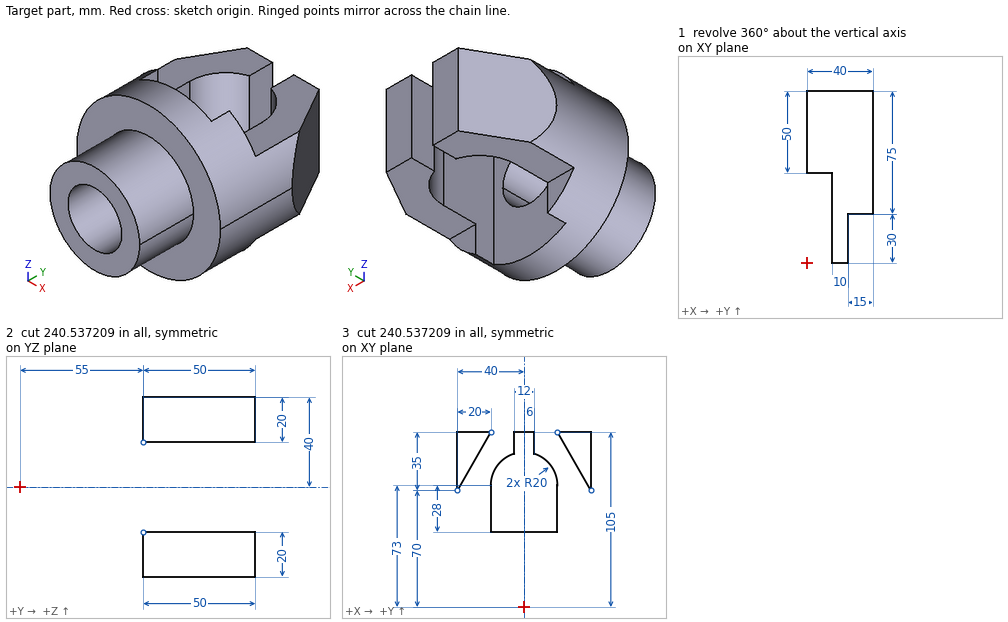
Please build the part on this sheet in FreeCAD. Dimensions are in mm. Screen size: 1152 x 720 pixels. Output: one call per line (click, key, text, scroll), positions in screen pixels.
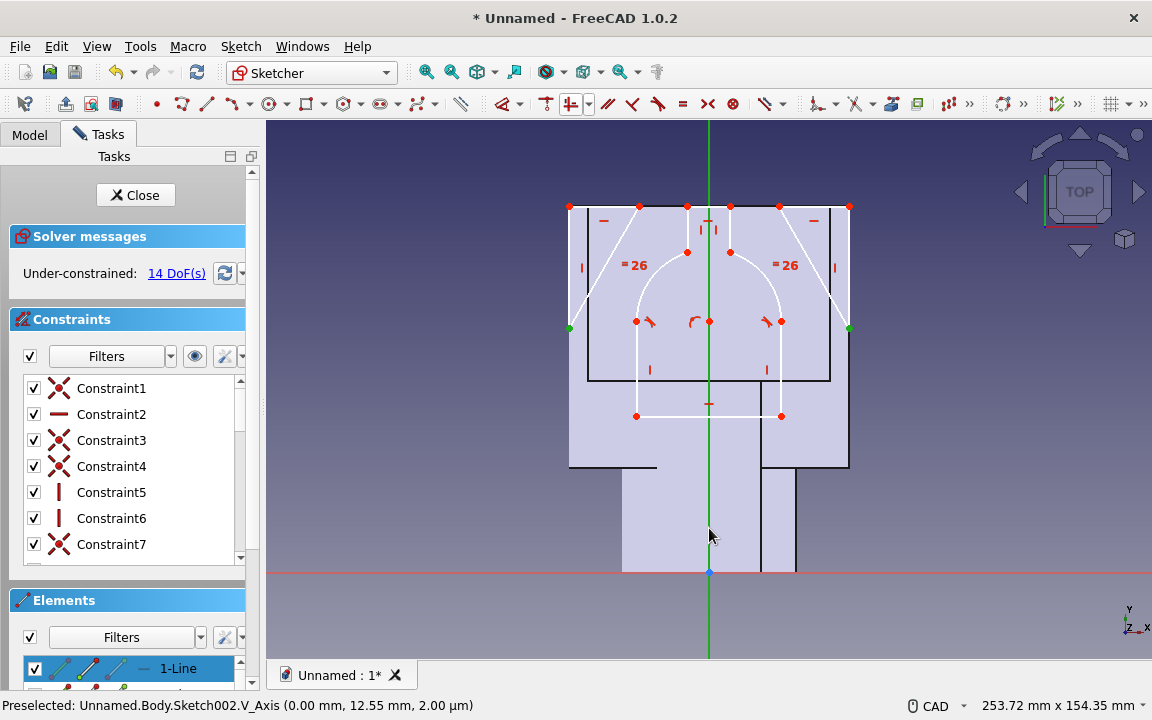
click(708, 104)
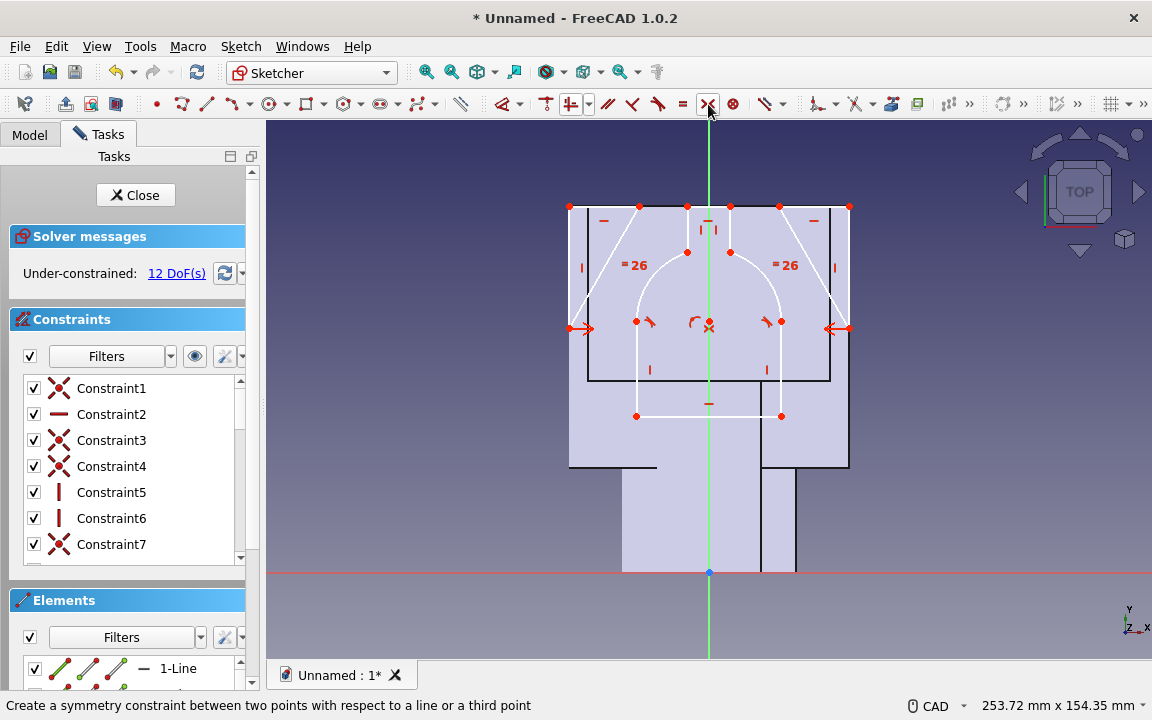
click(639, 207)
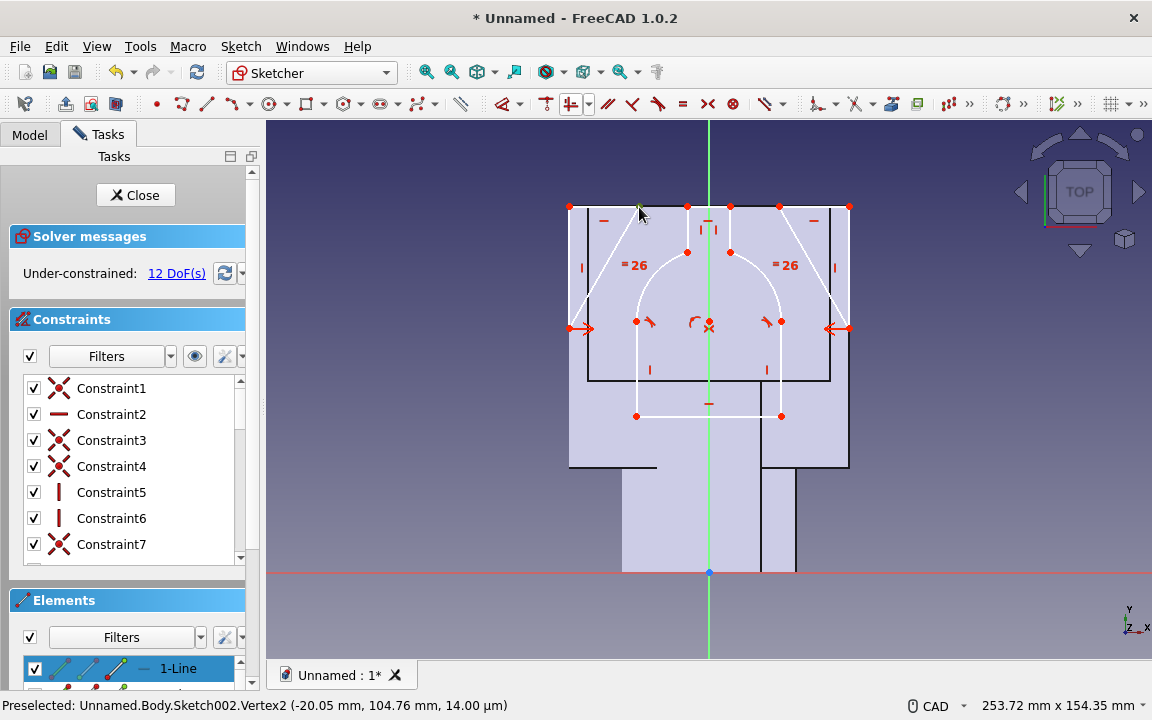
click(779, 207)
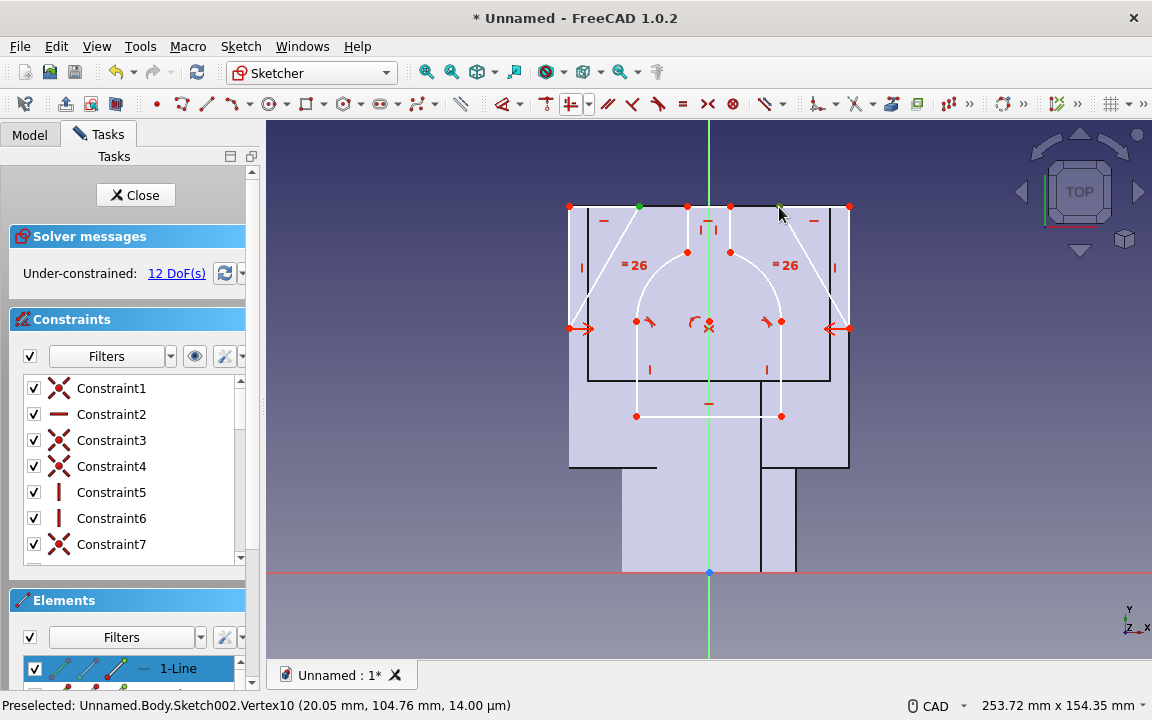
click(709, 528)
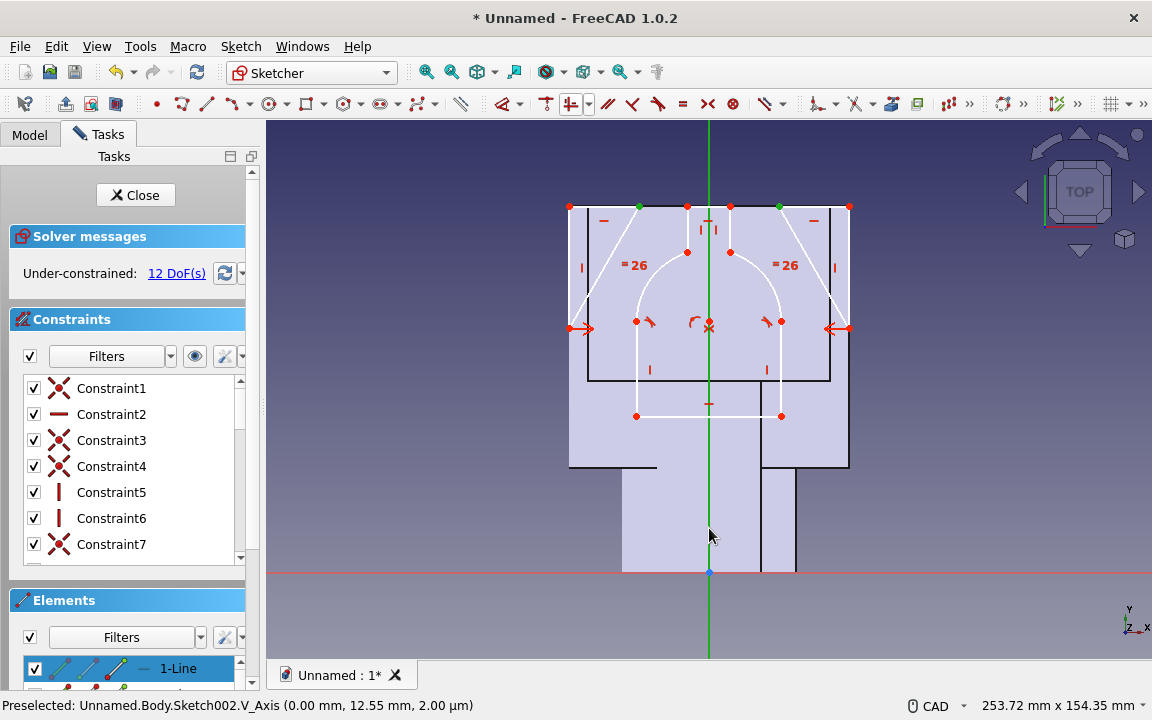
click(708, 104)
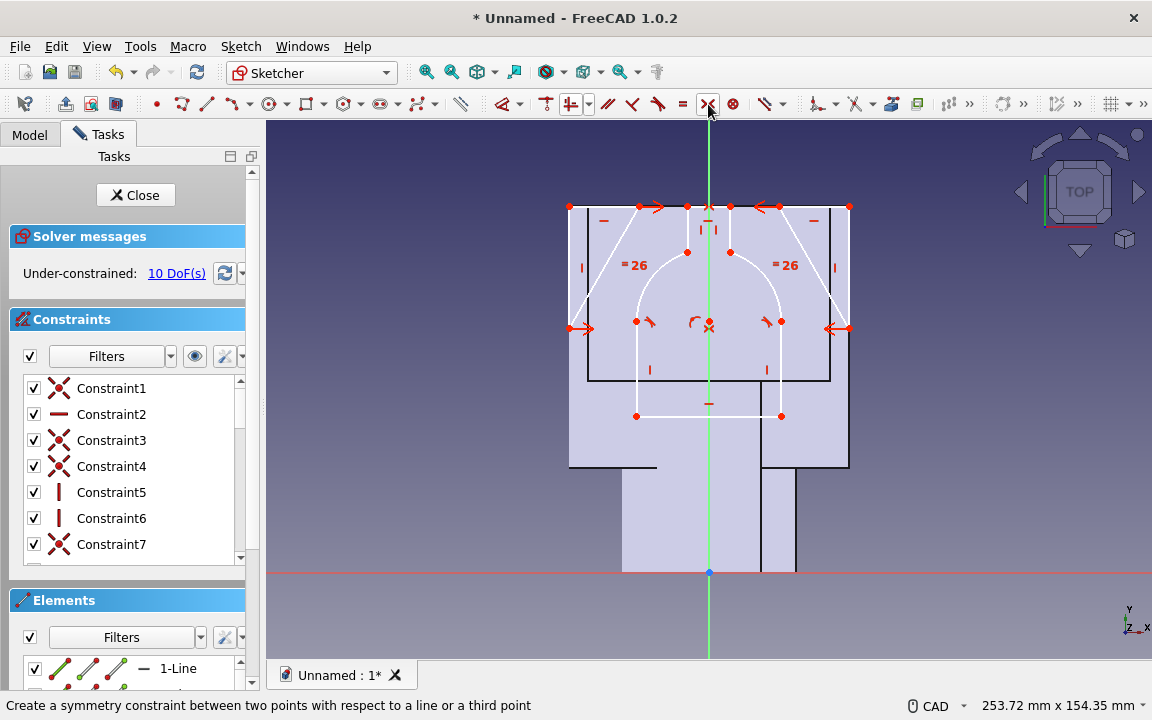
click(502, 104)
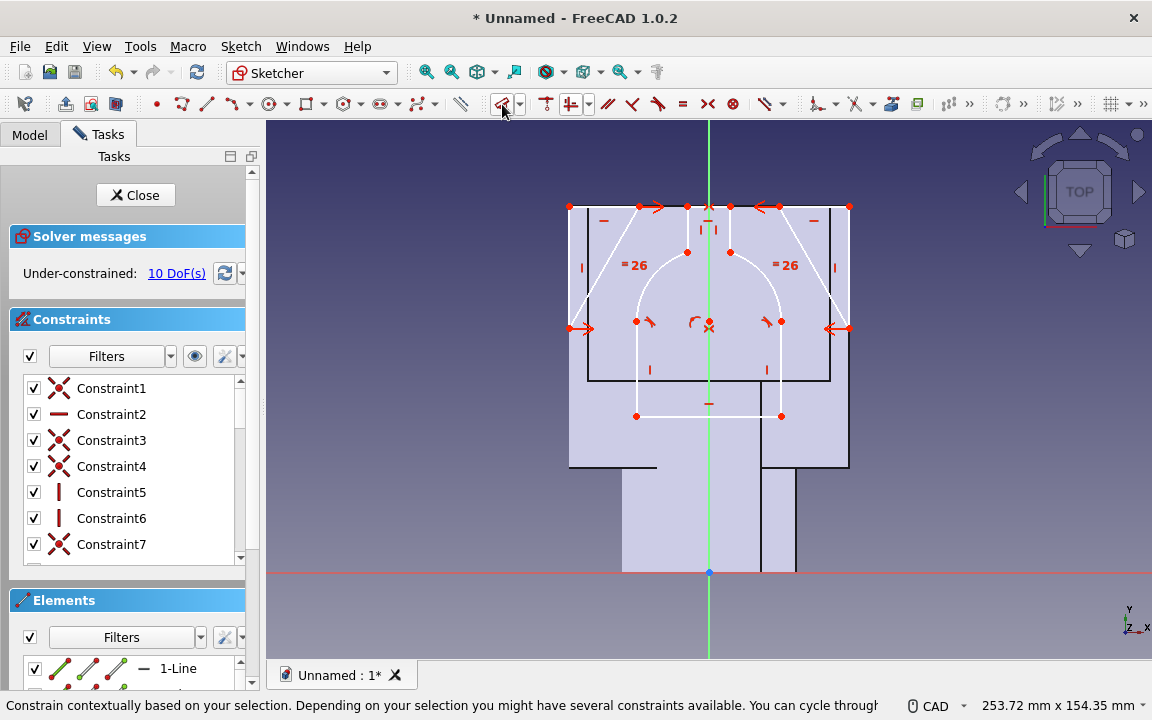
click(664, 265)
click(644, 240)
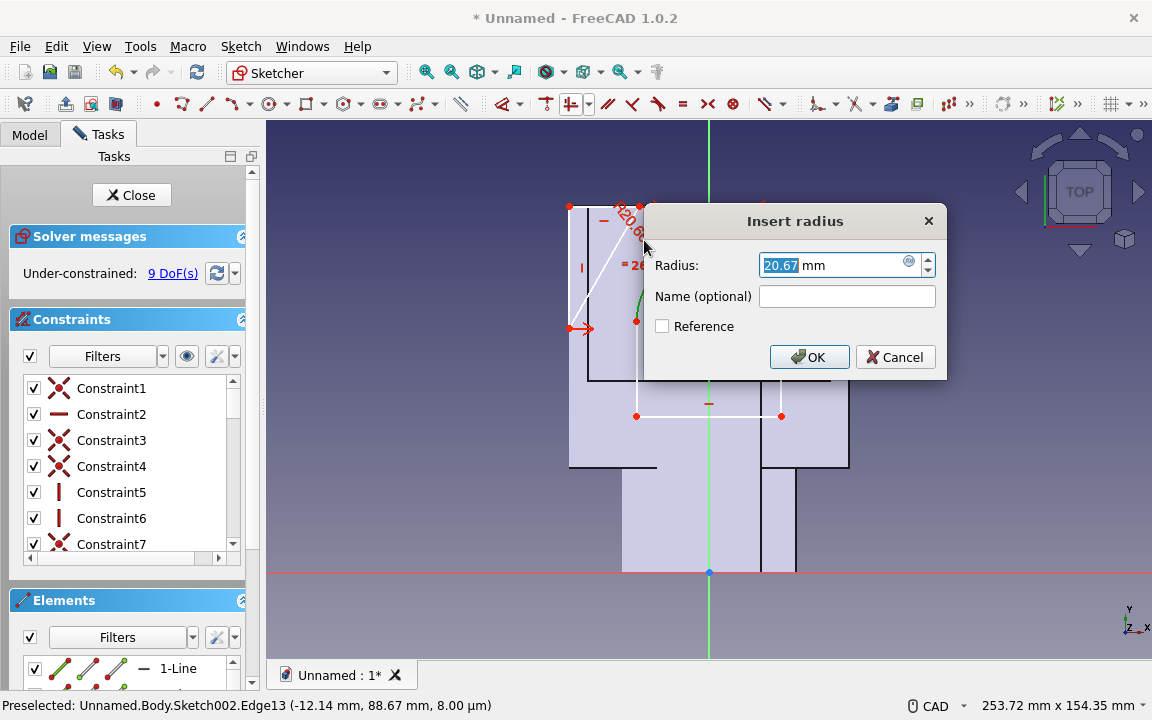
text(20)
key(Return)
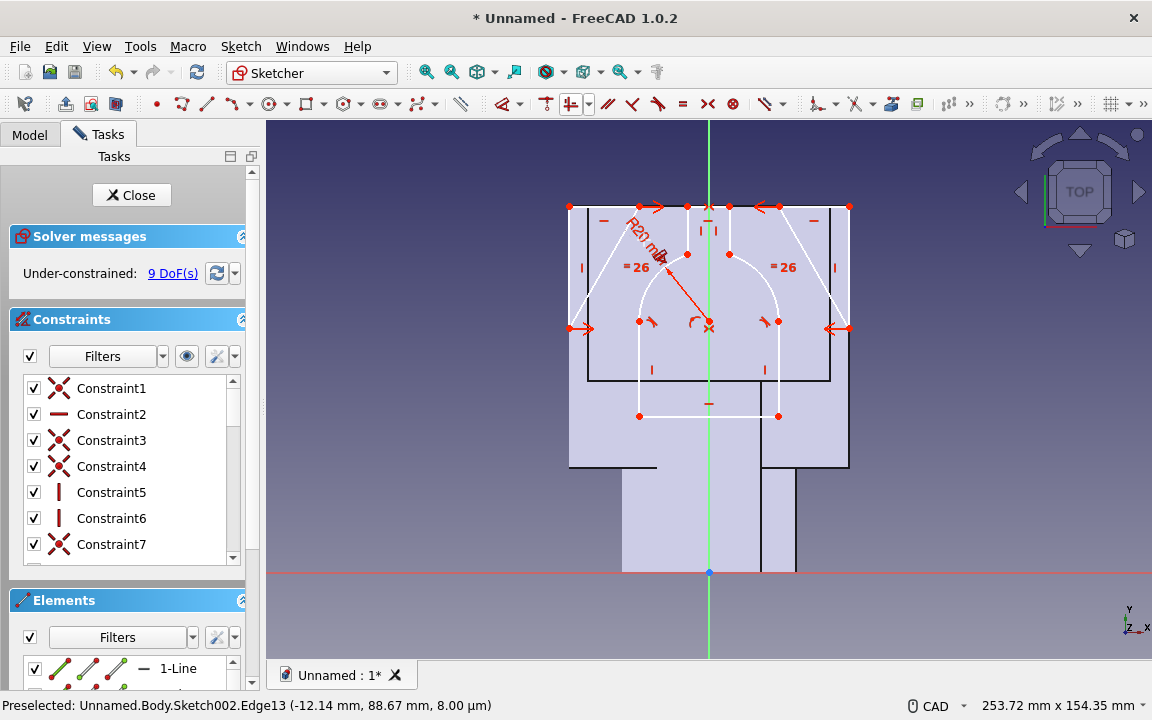
click(618, 207)
click(604, 173)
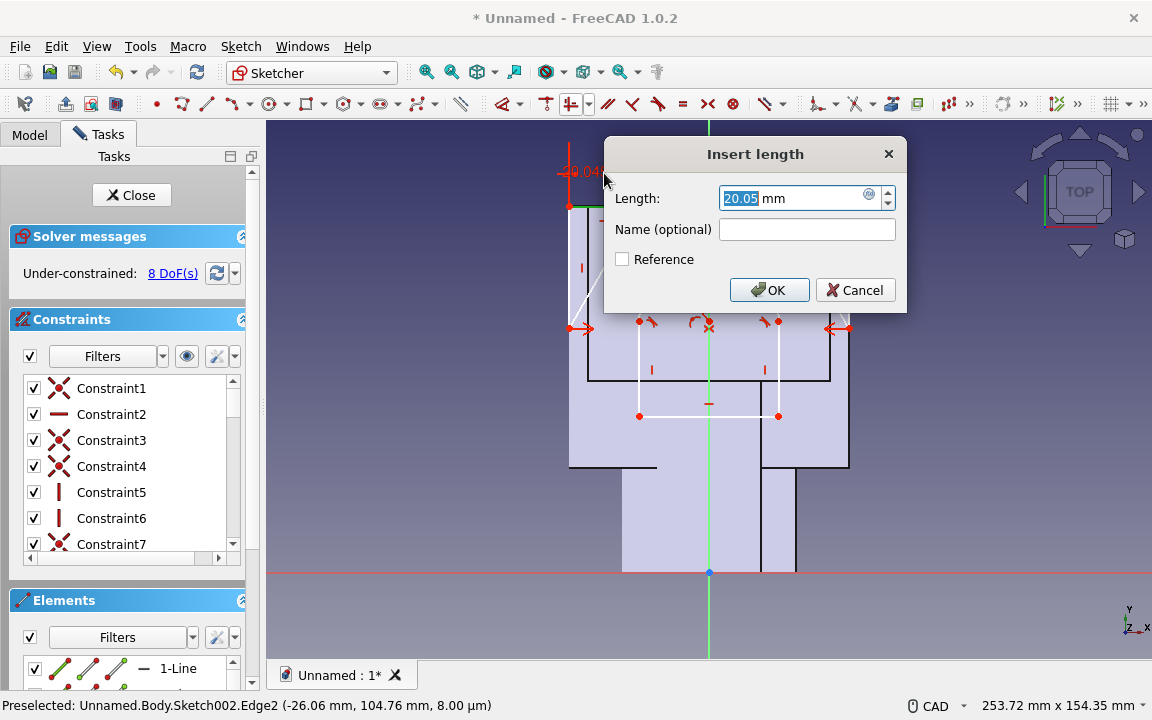
text(20)
key(Return)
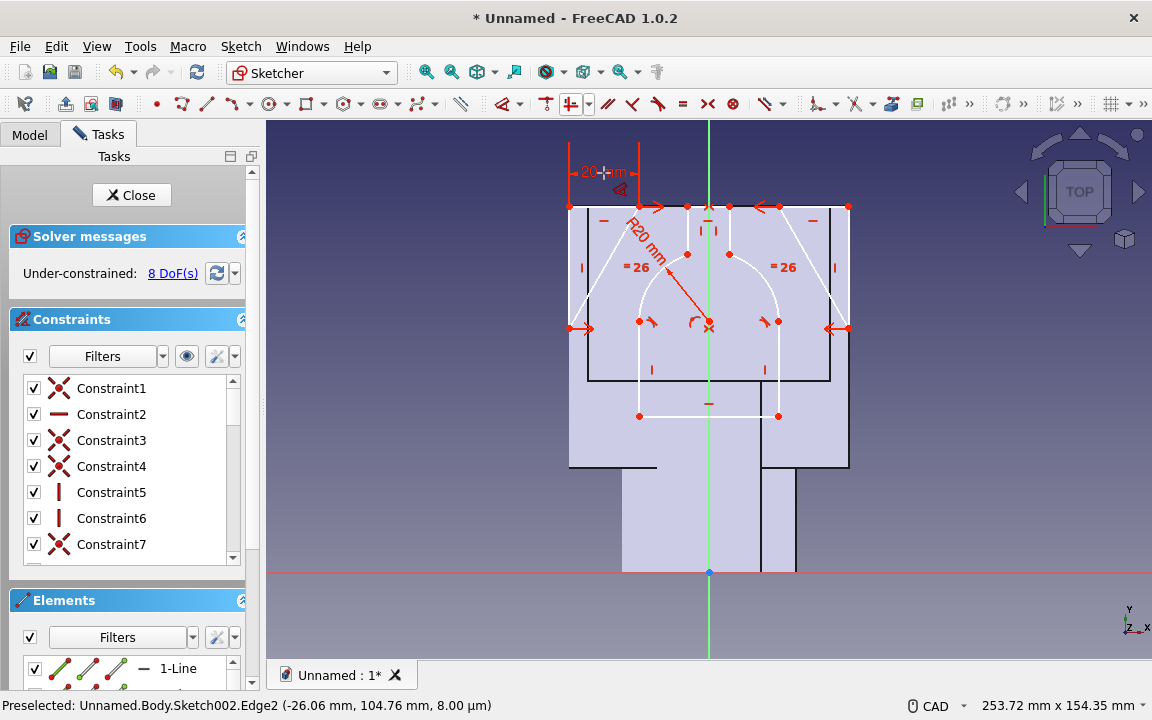
click(569, 244)
click(535, 268)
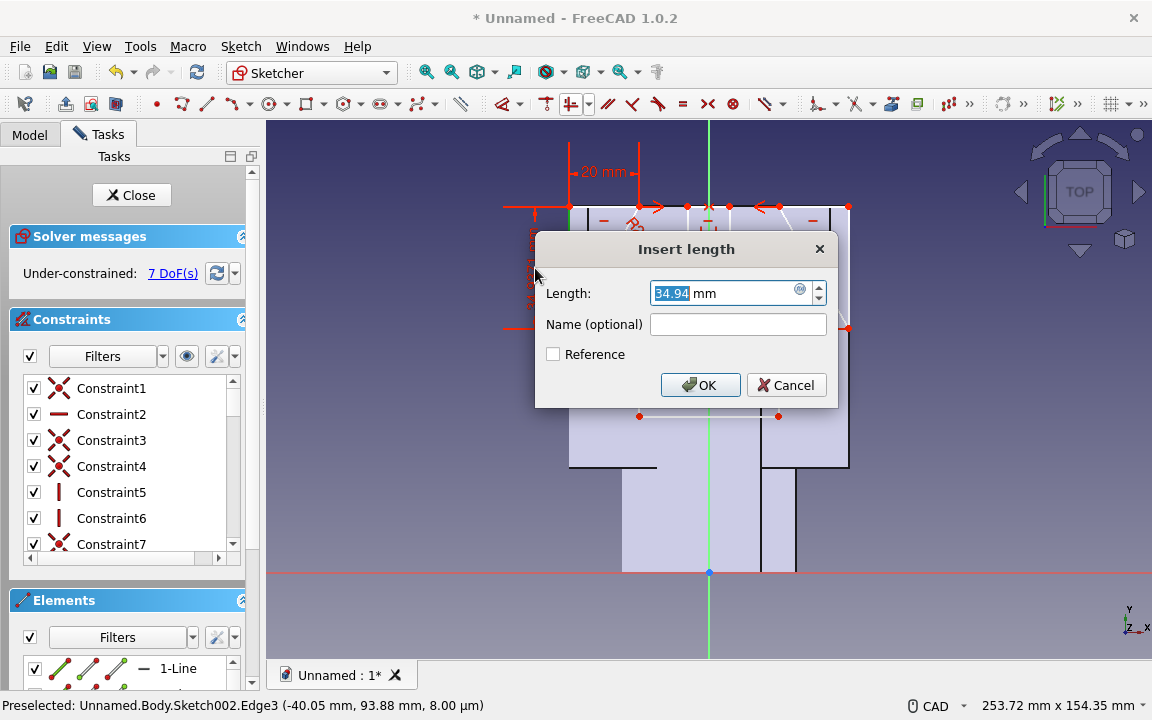
text(35)
key(Return)